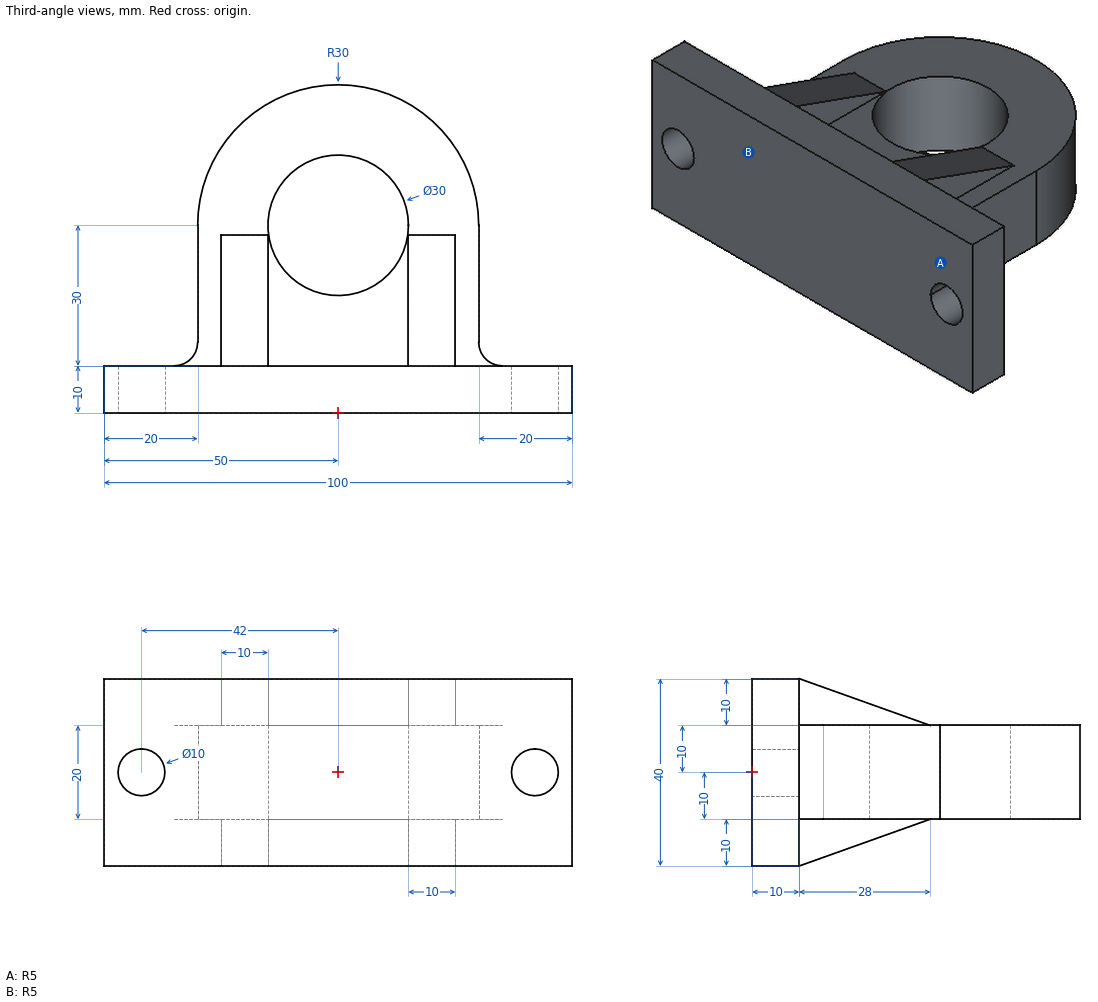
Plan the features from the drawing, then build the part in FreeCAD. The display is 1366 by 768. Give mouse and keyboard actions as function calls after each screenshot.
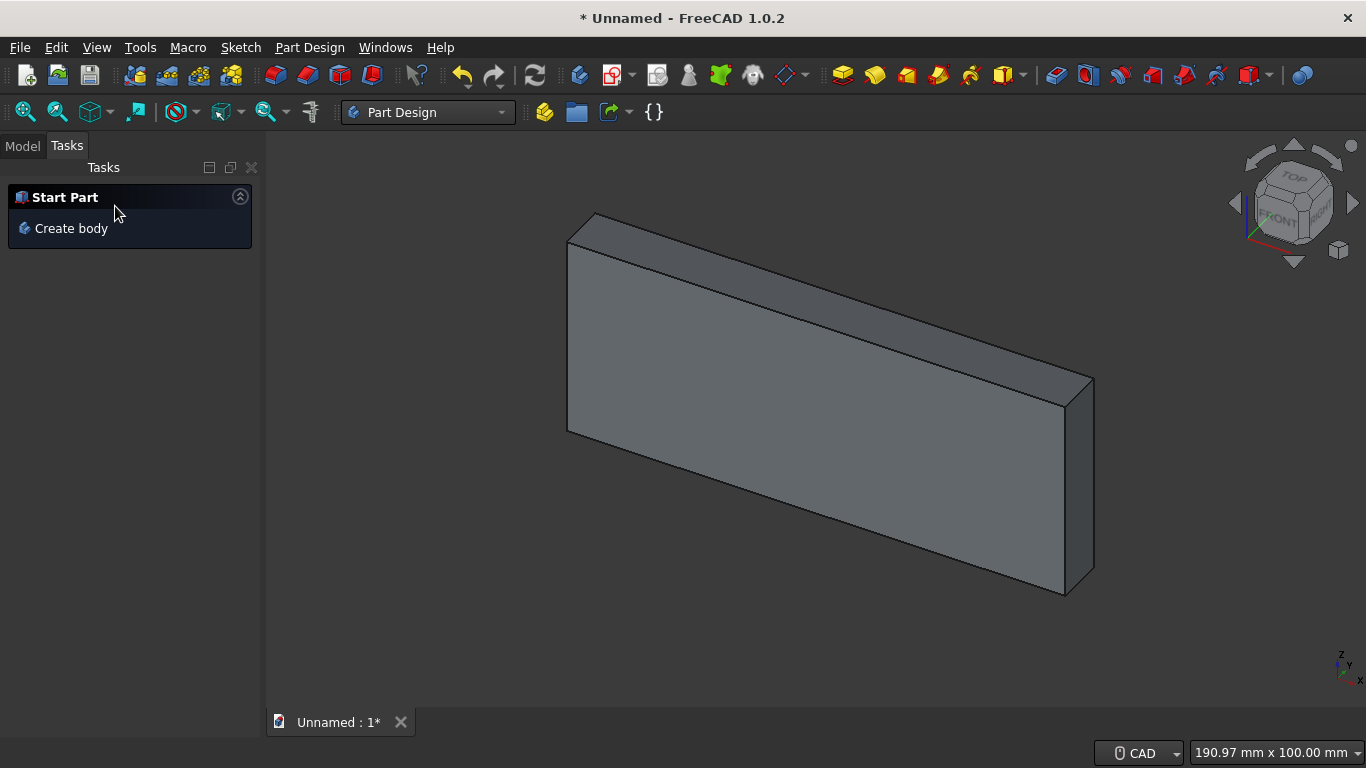
click(612, 76)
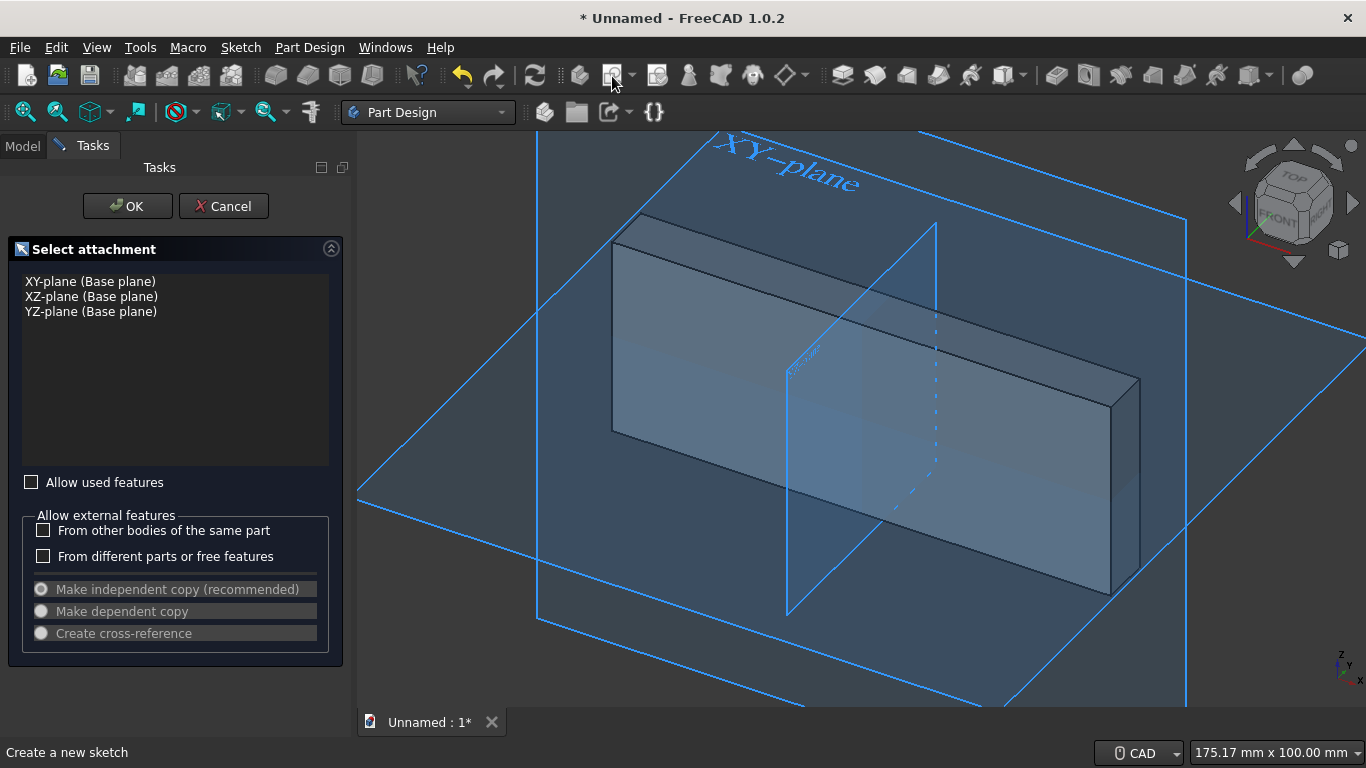
click(82, 282)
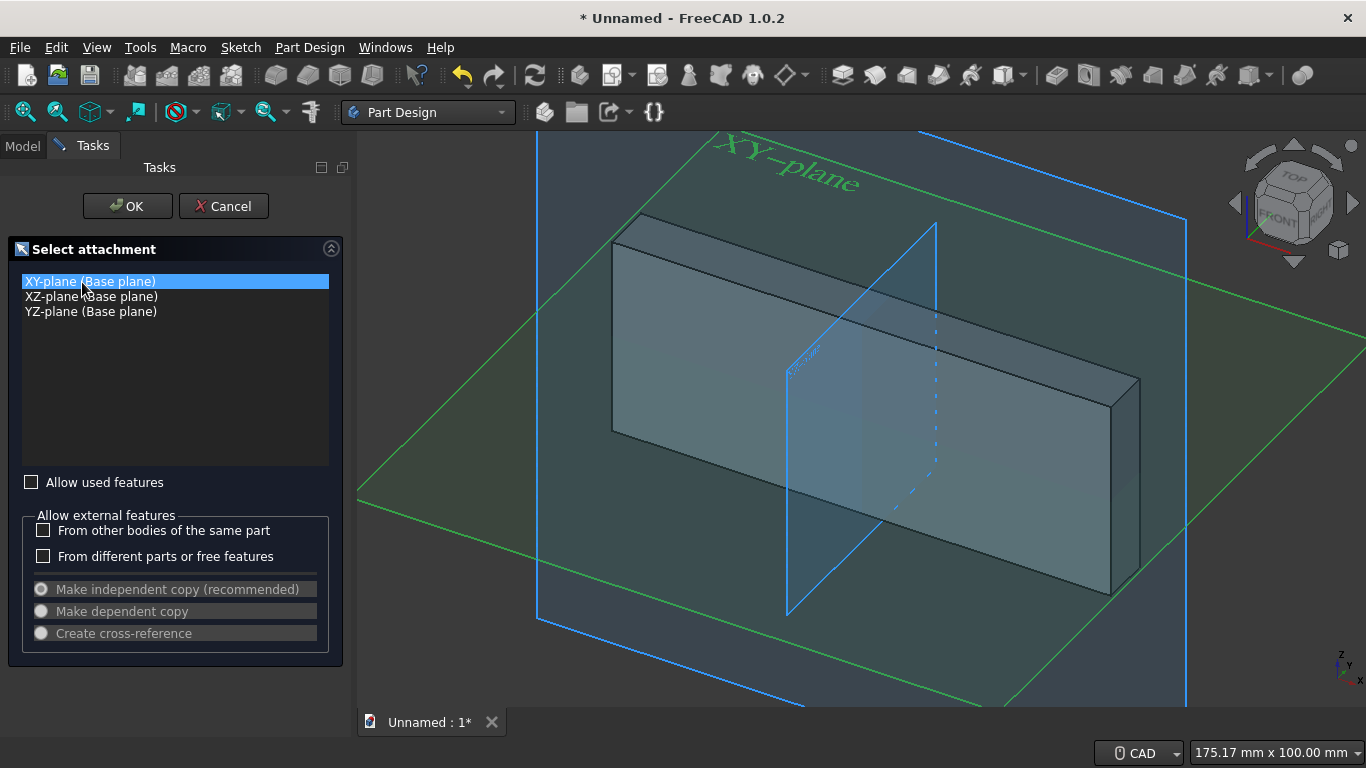
click(128, 206)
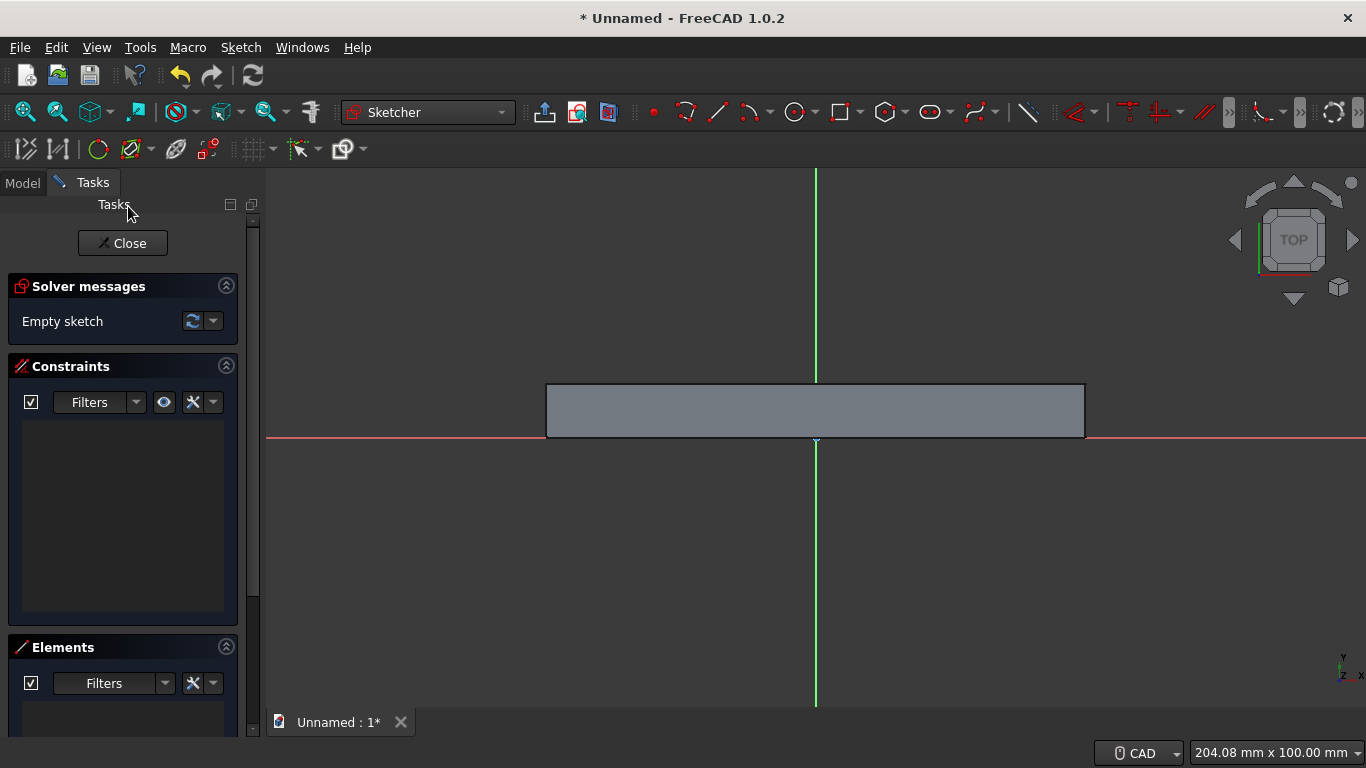
click(610, 112)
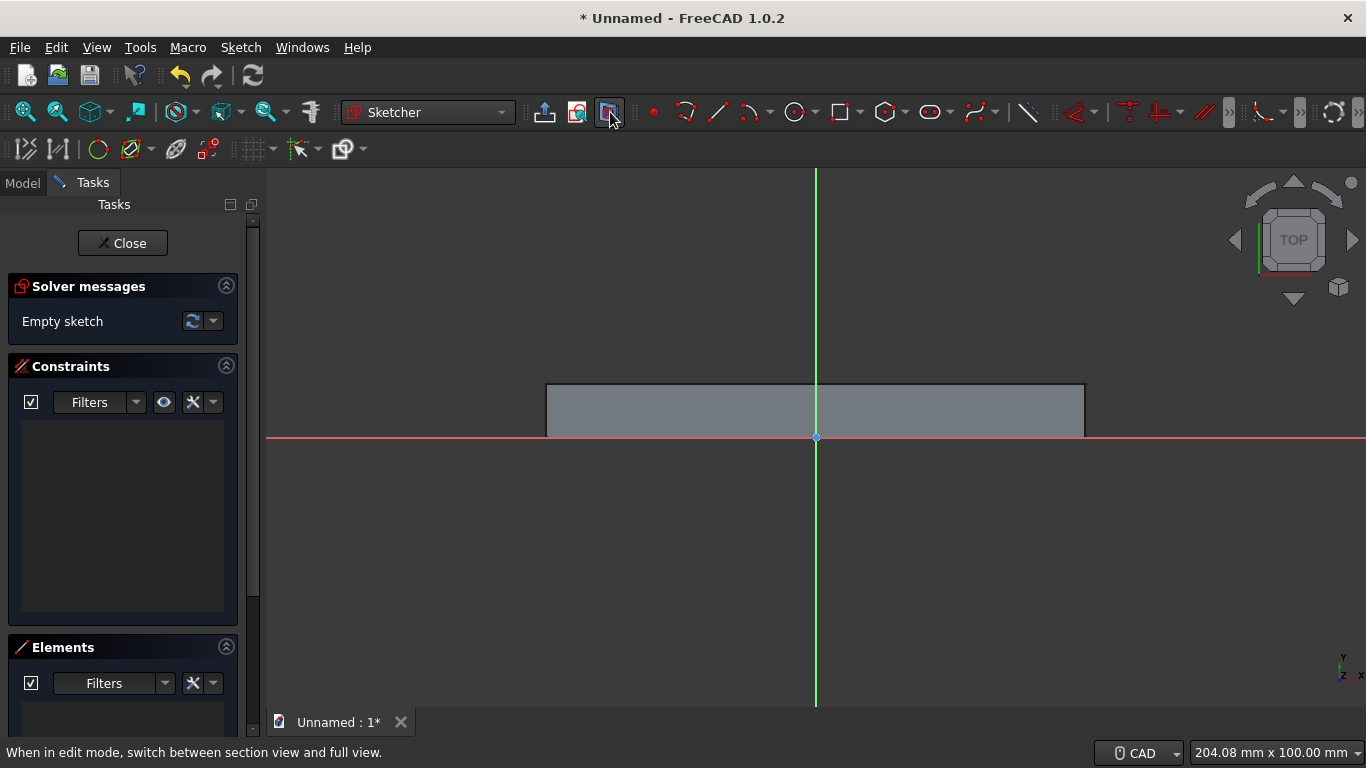
scroll(608, 679, down, 2)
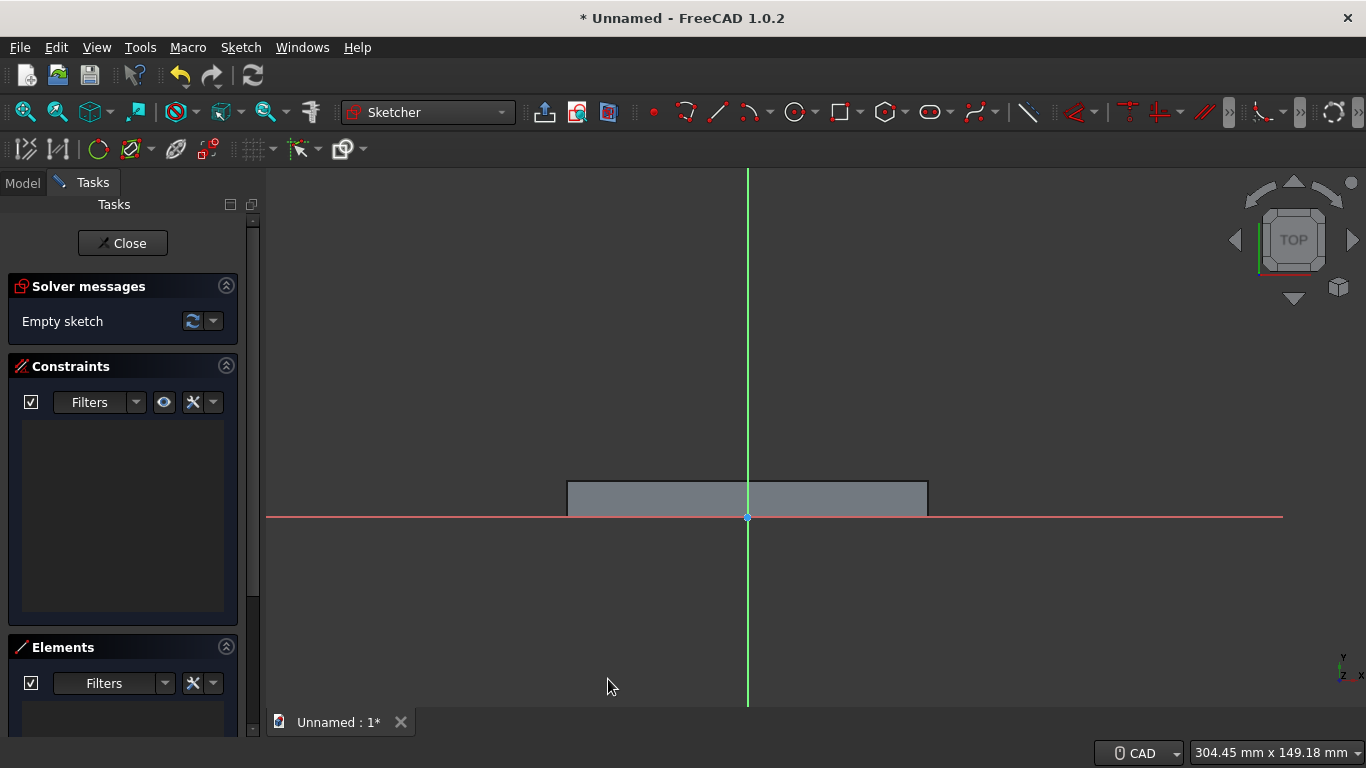
key(g)
key(m)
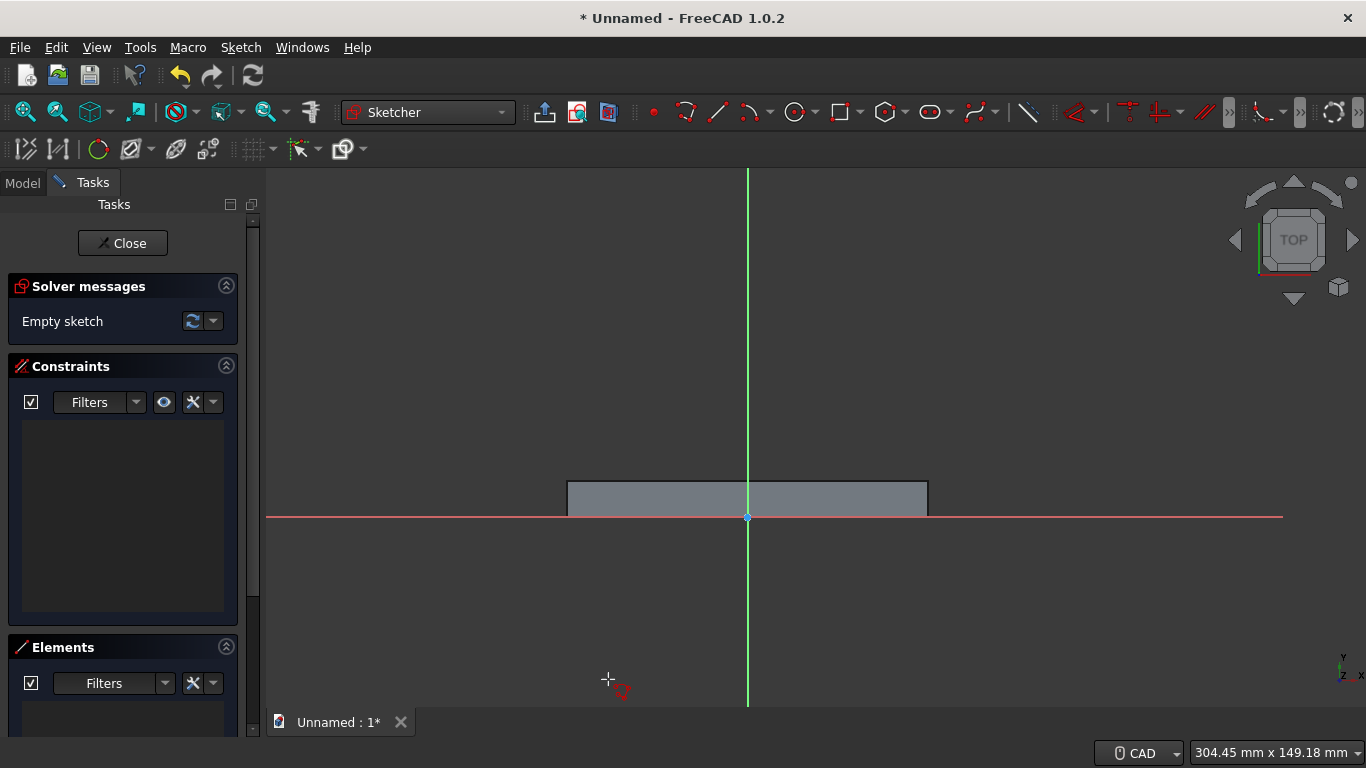
click(639, 373)
click(639, 481)
click(567, 481)
click(567, 517)
click(928, 508)
click(928, 481)
click(856, 481)
click(856, 373)
right_click(856, 373)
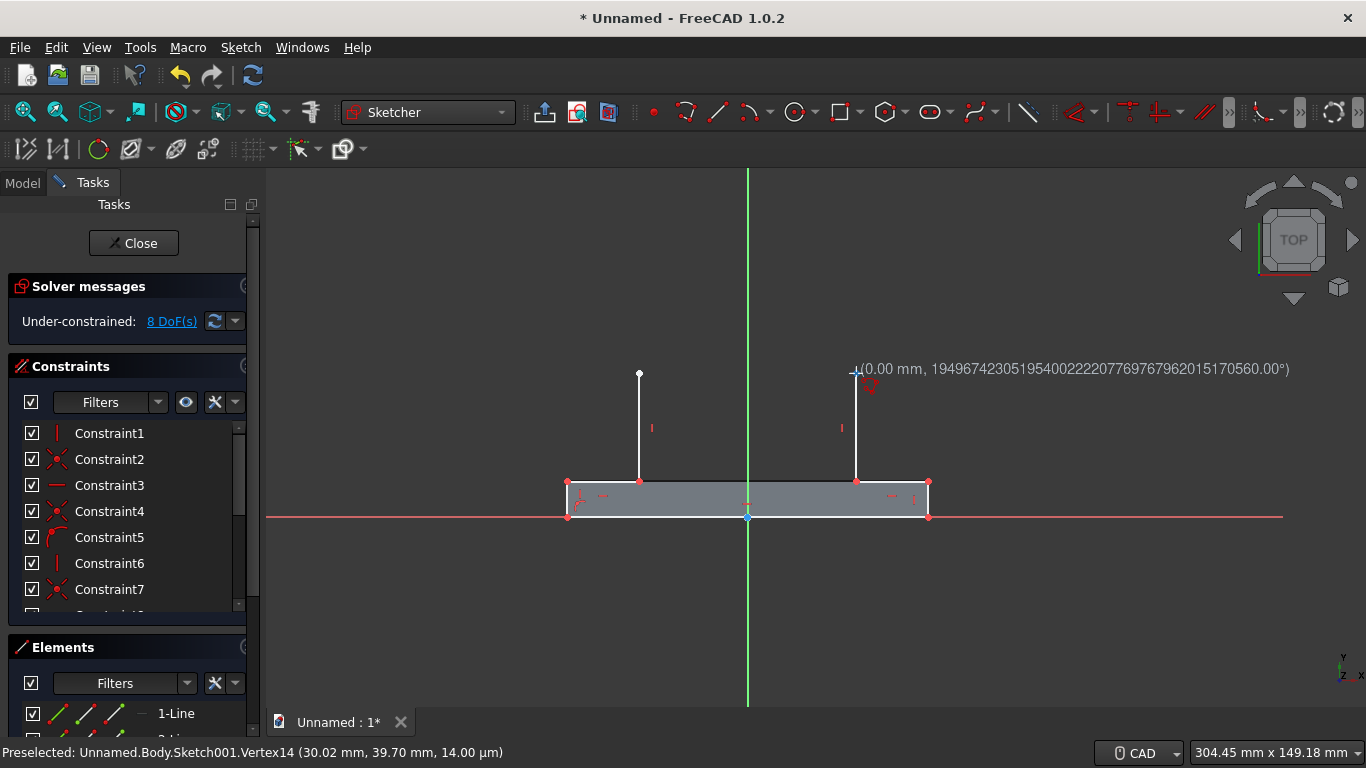
click(772, 112)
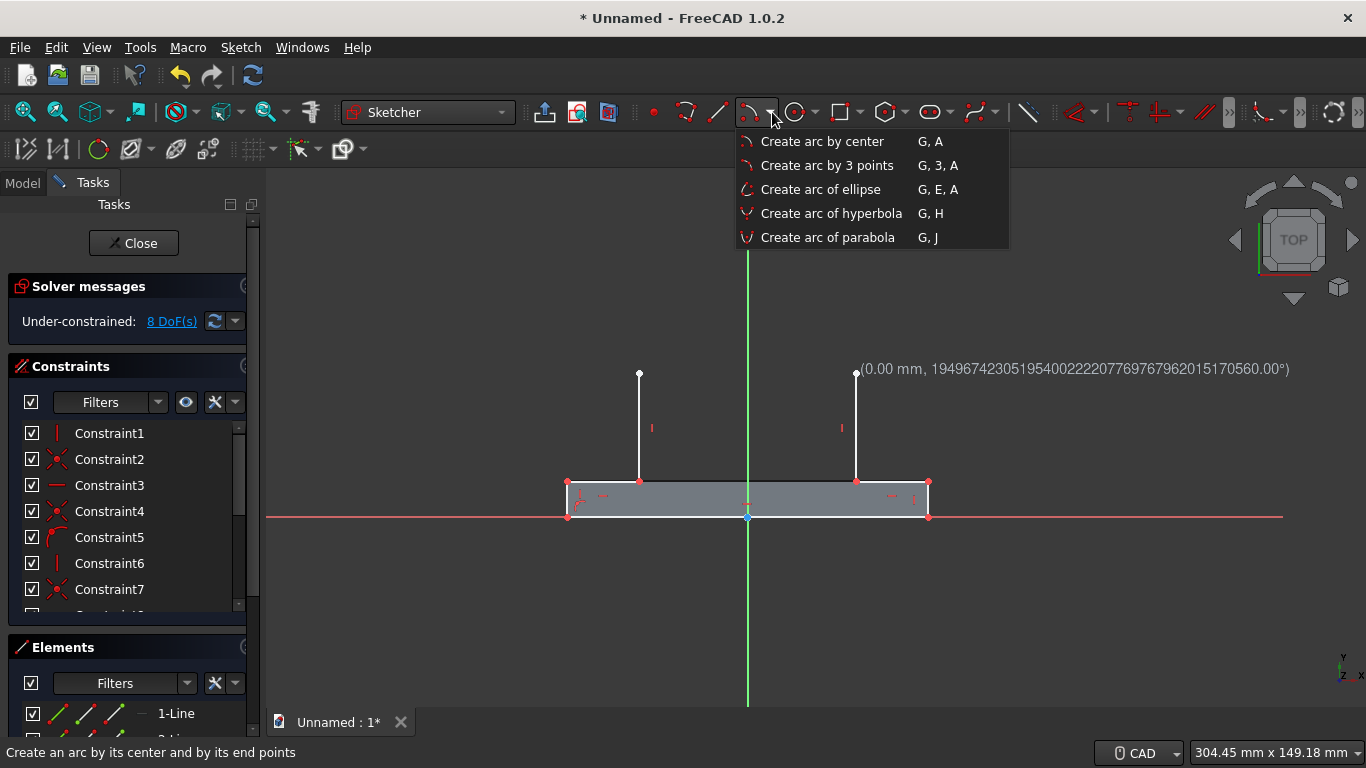
click(872, 165)